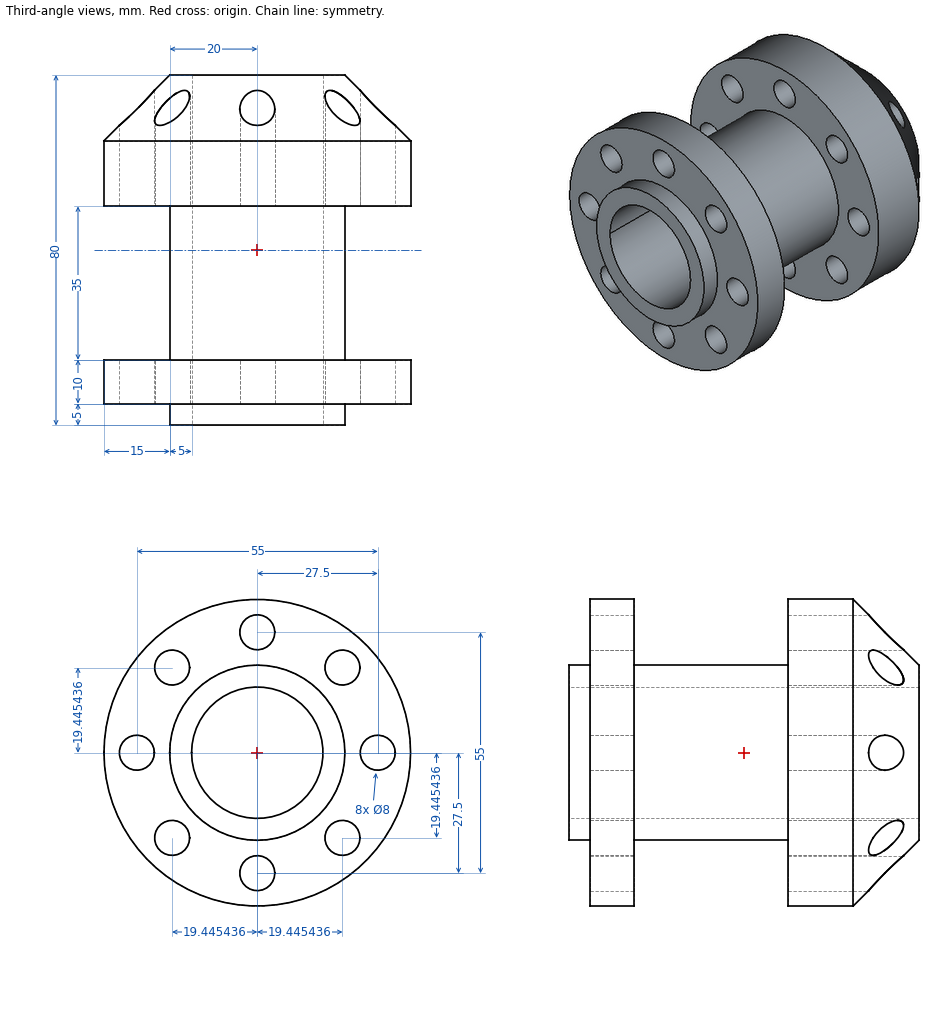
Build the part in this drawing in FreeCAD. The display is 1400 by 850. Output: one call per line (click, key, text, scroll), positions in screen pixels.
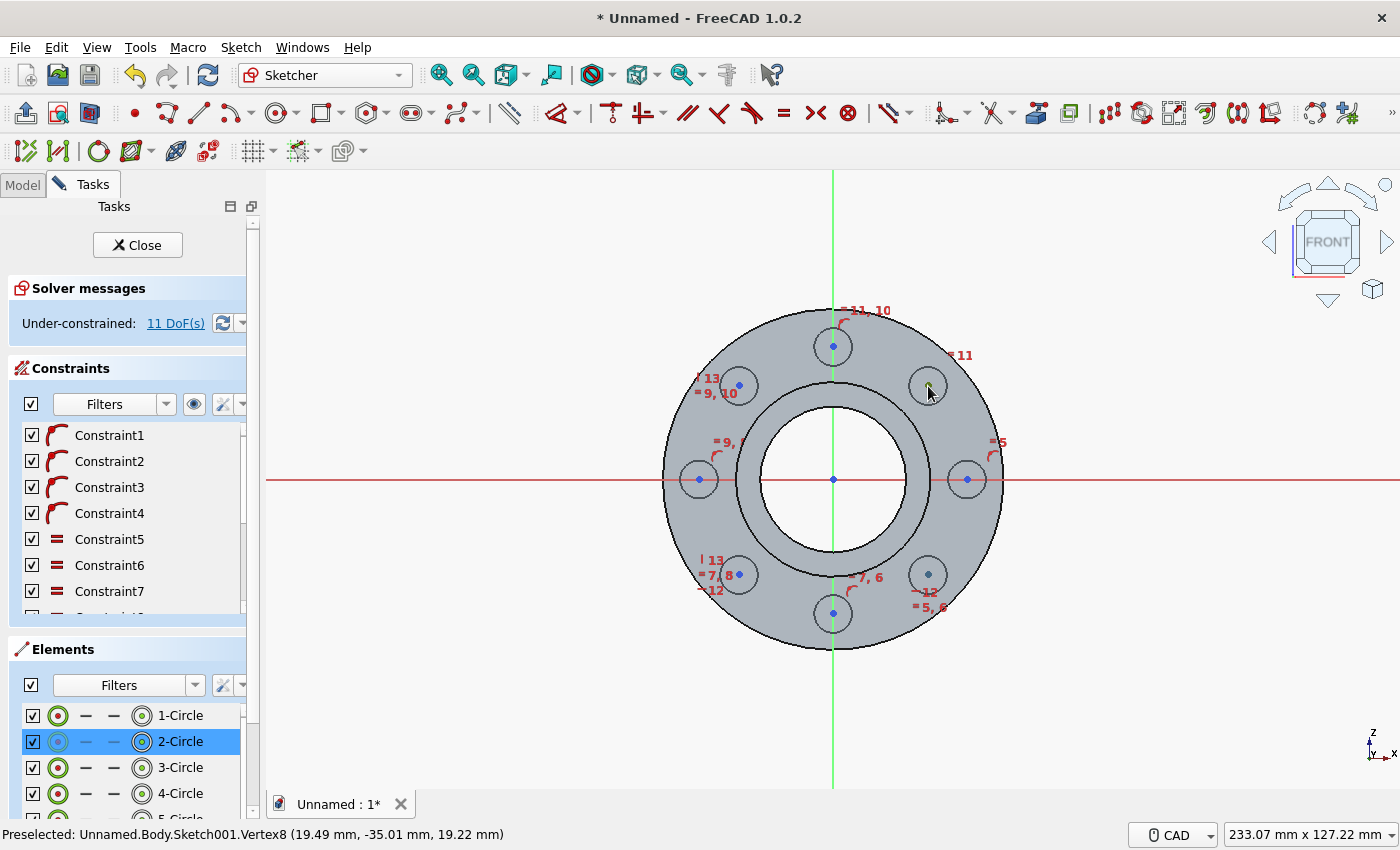
key(v)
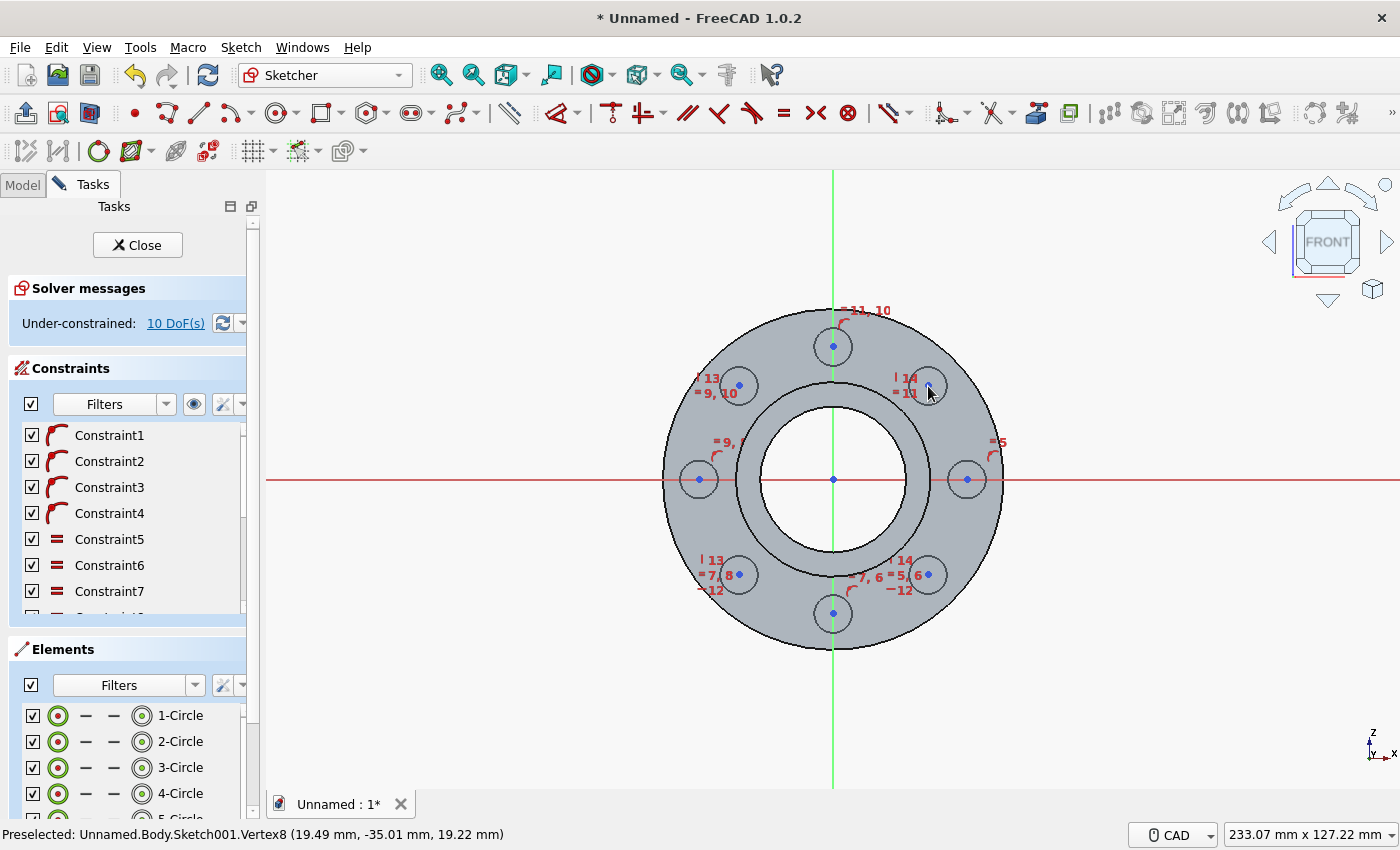
click(739, 386)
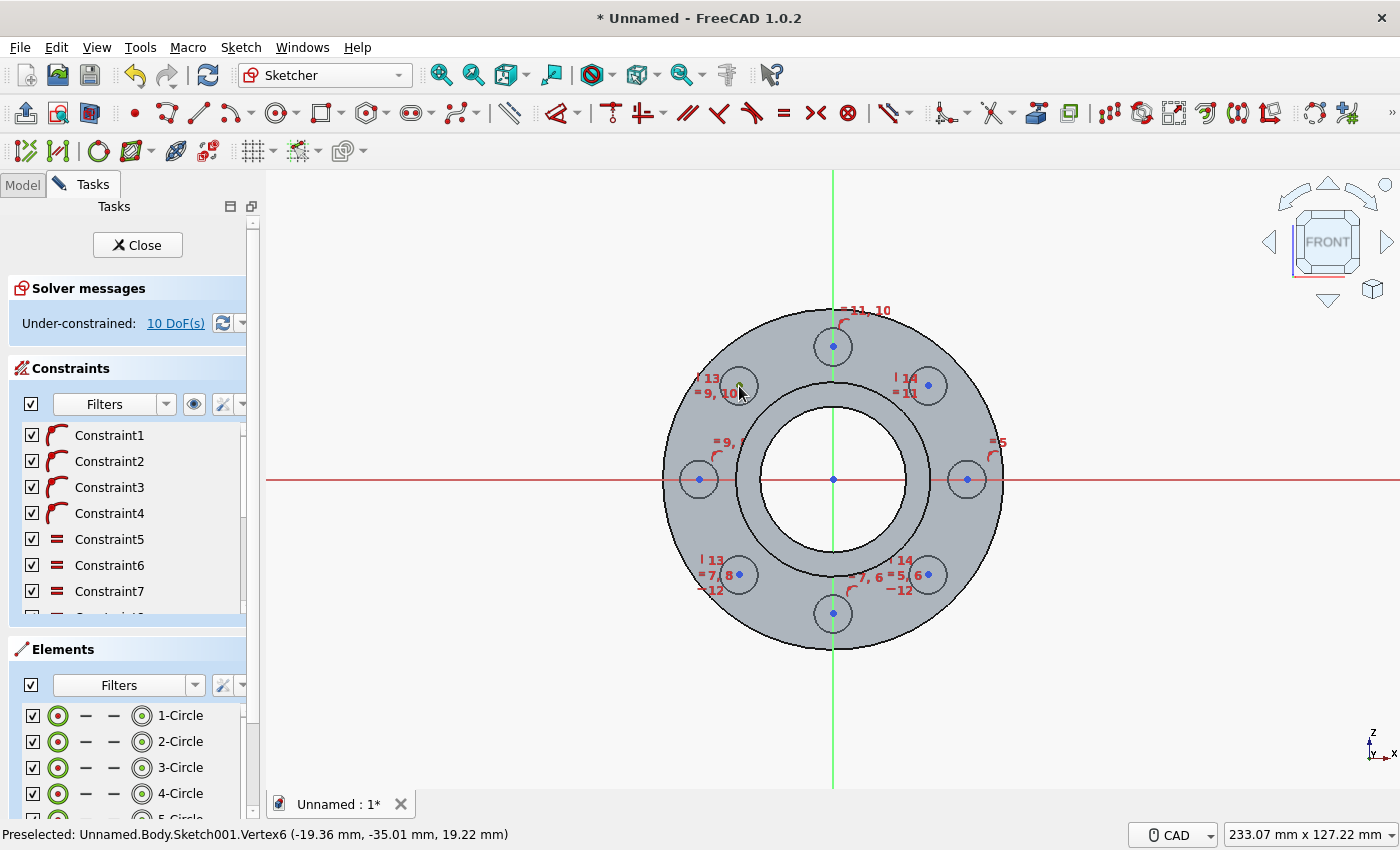
click(928, 386)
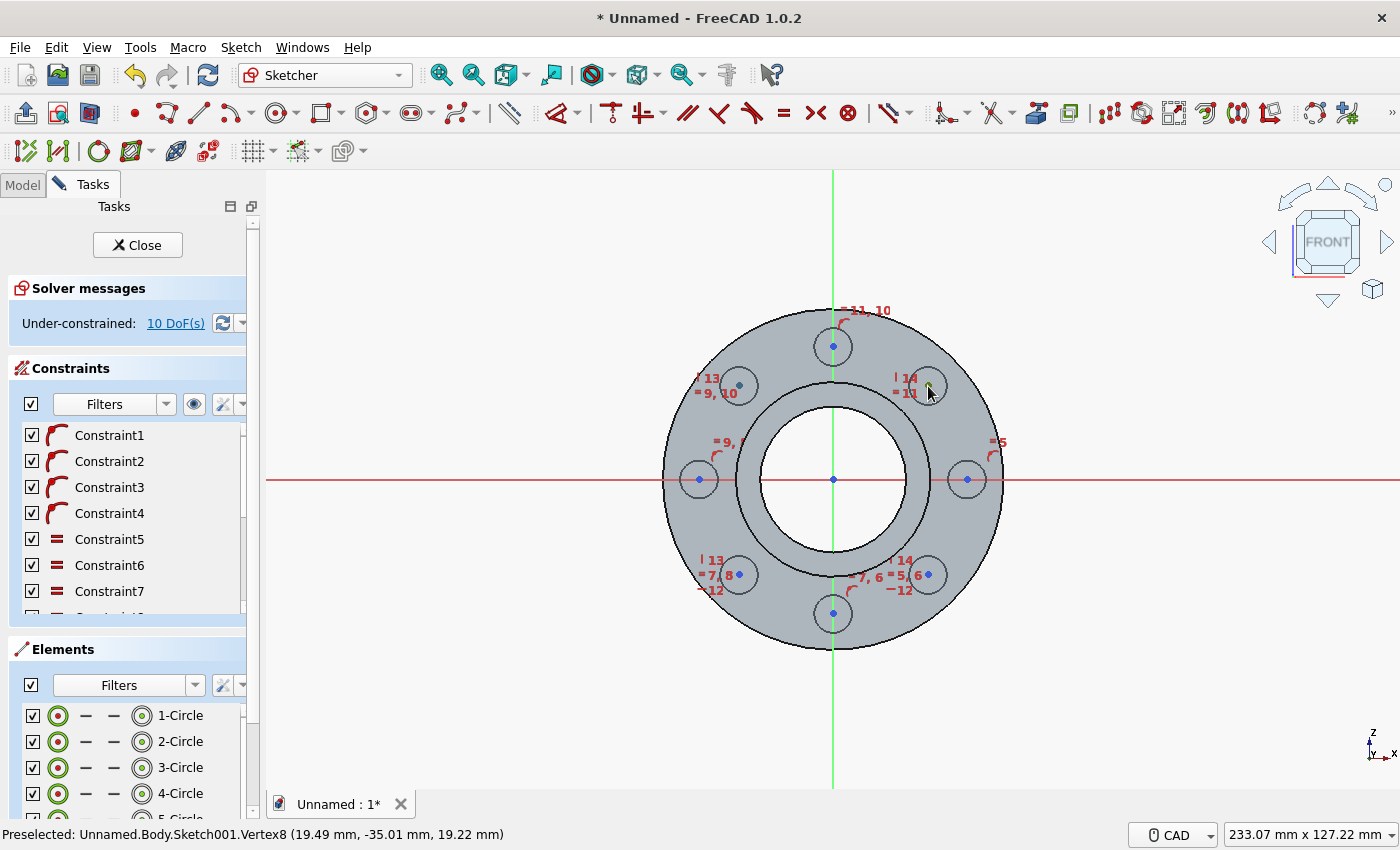
key(h)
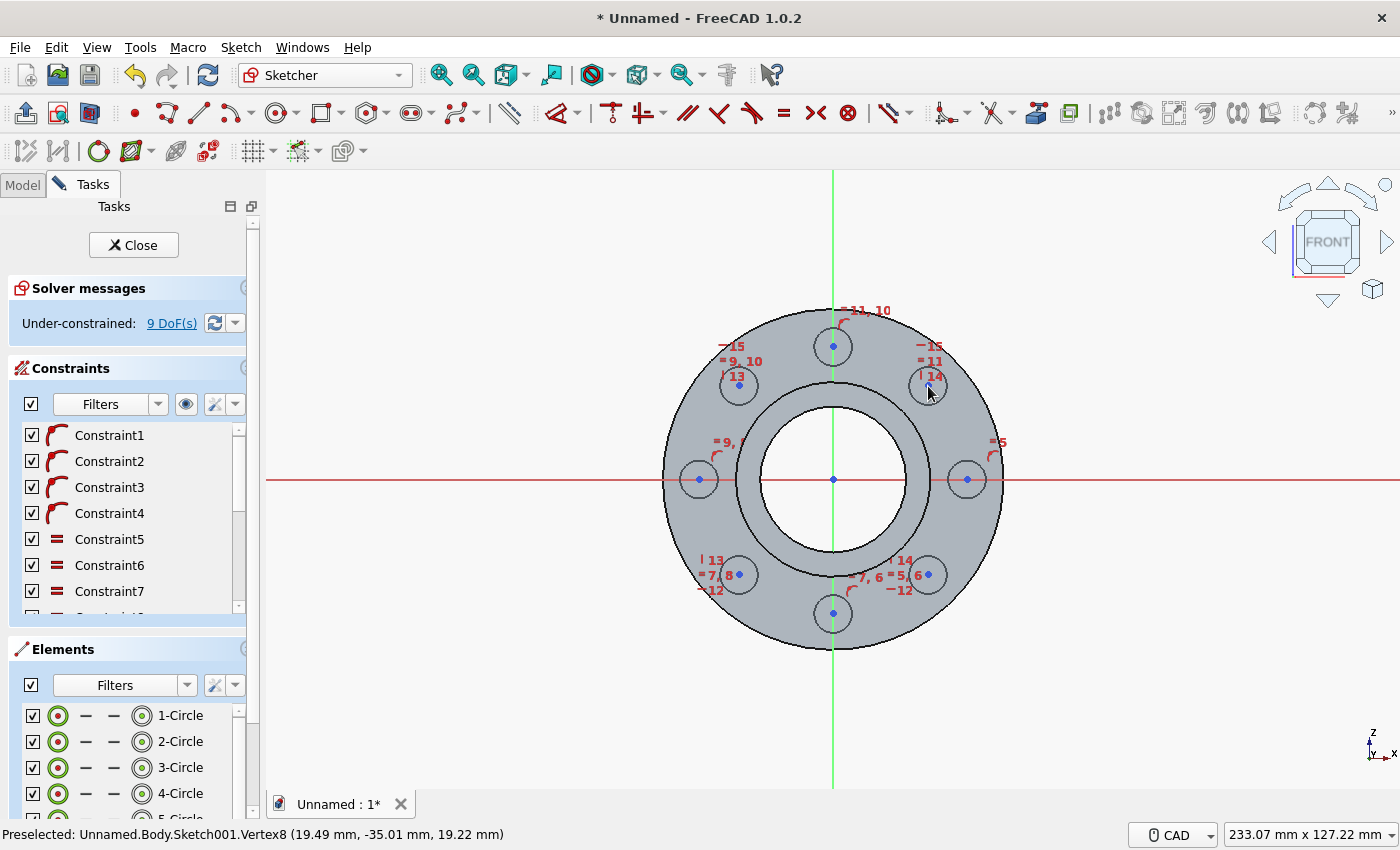
key(d)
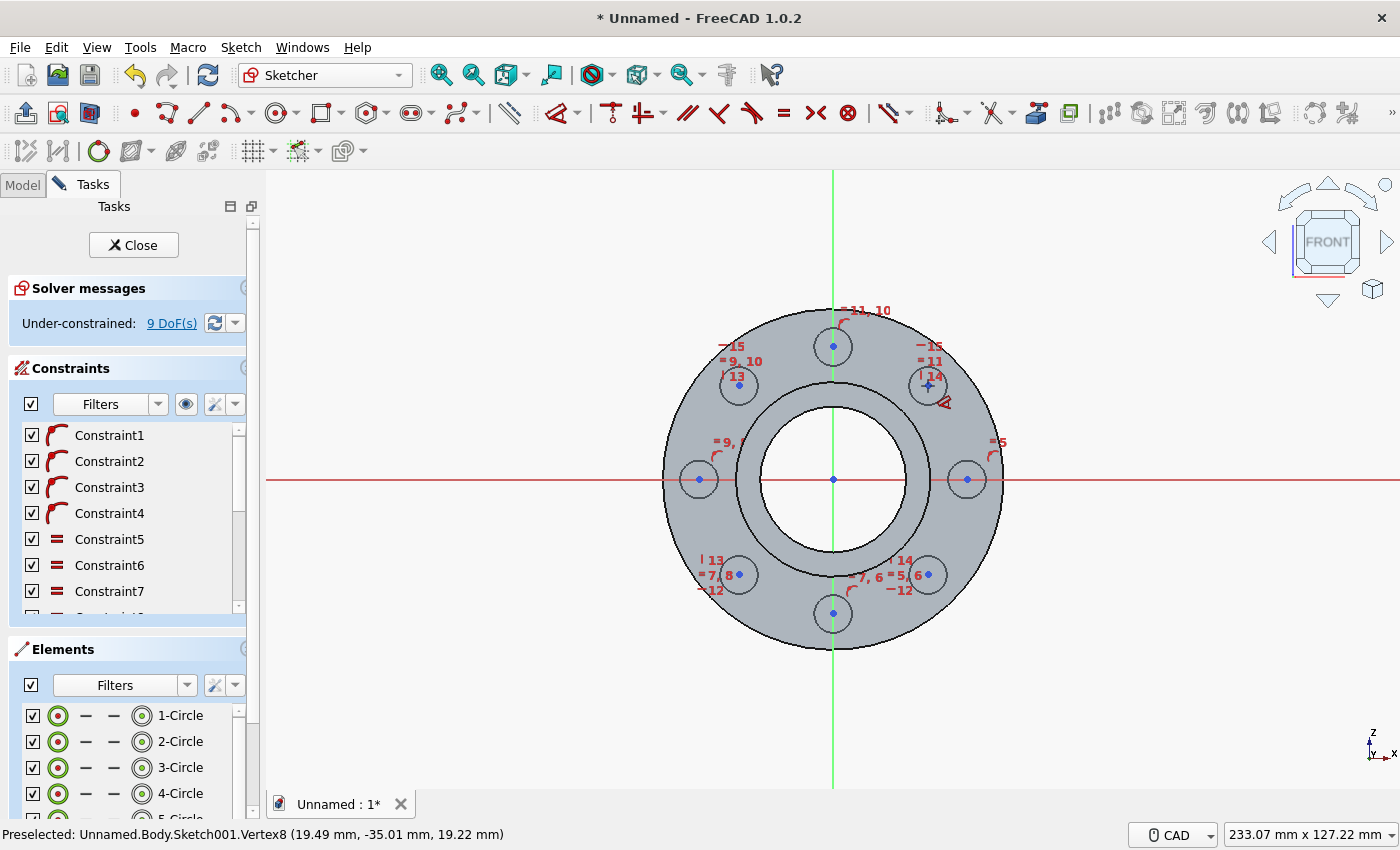
click(980, 466)
click(1002, 443)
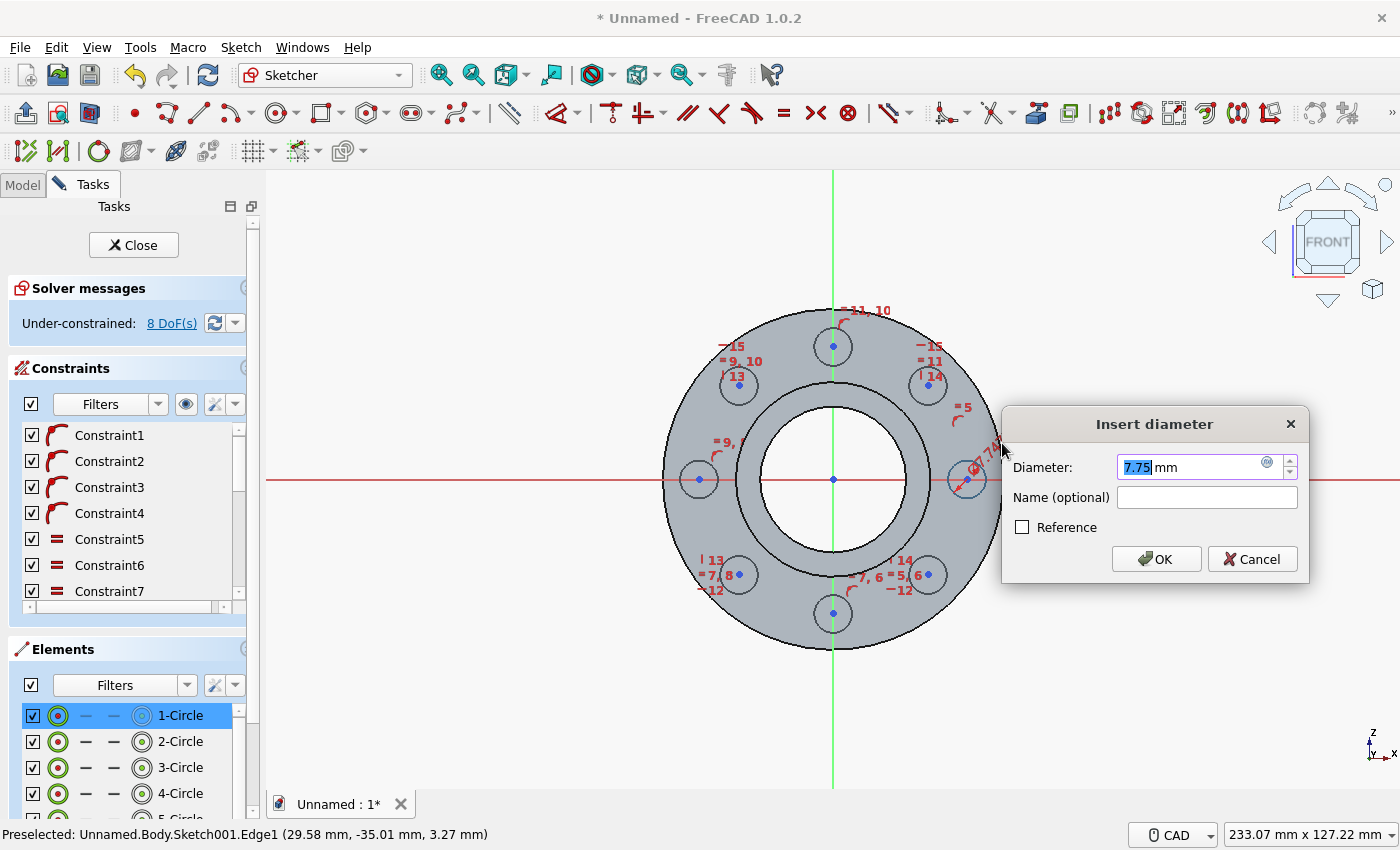
text(8)
key(Return)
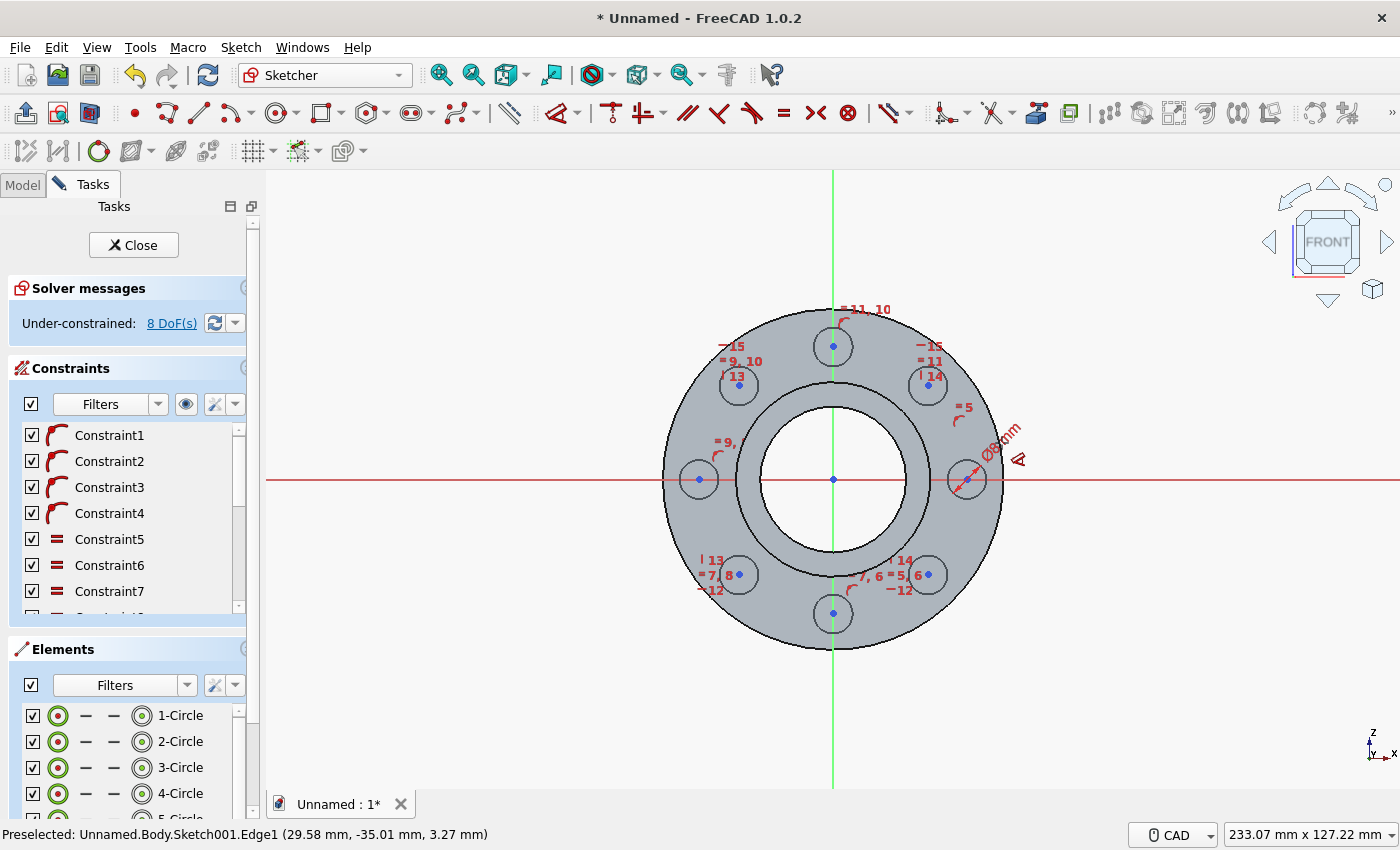
click(967, 480)